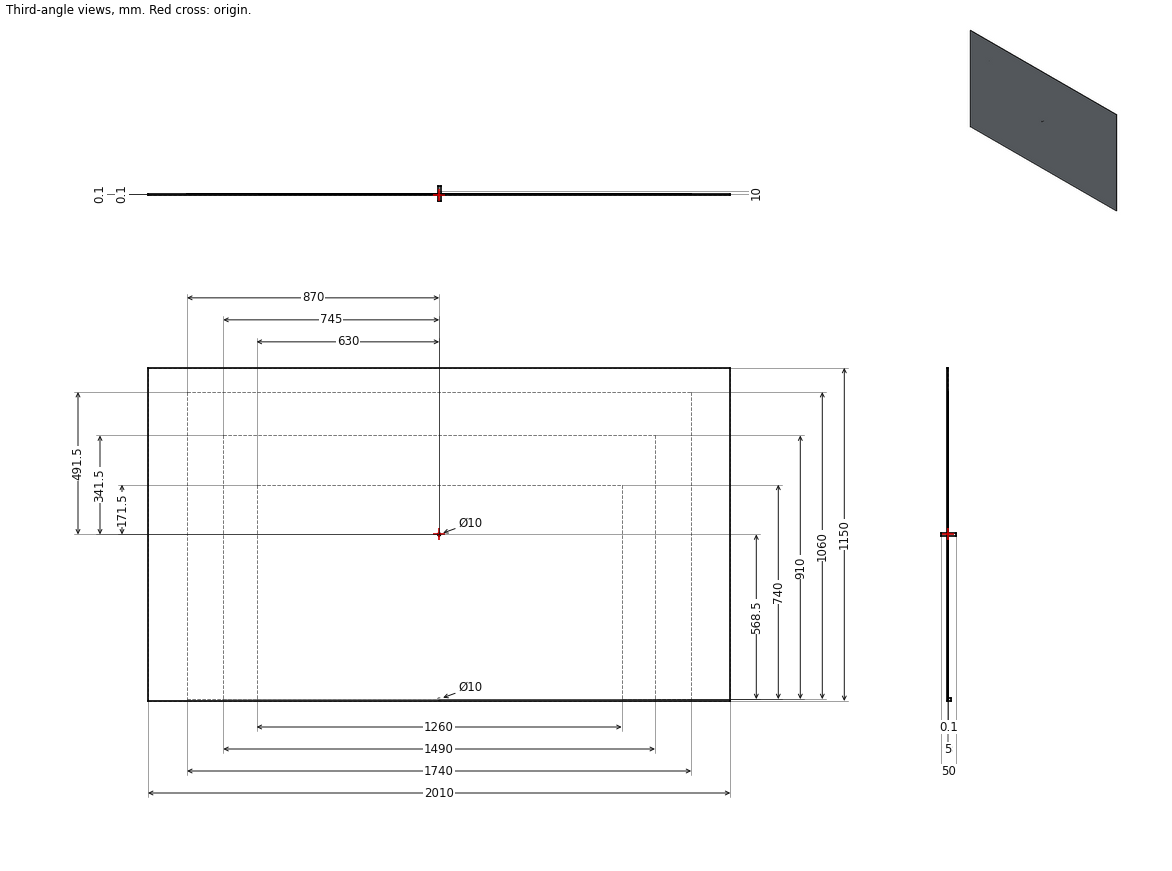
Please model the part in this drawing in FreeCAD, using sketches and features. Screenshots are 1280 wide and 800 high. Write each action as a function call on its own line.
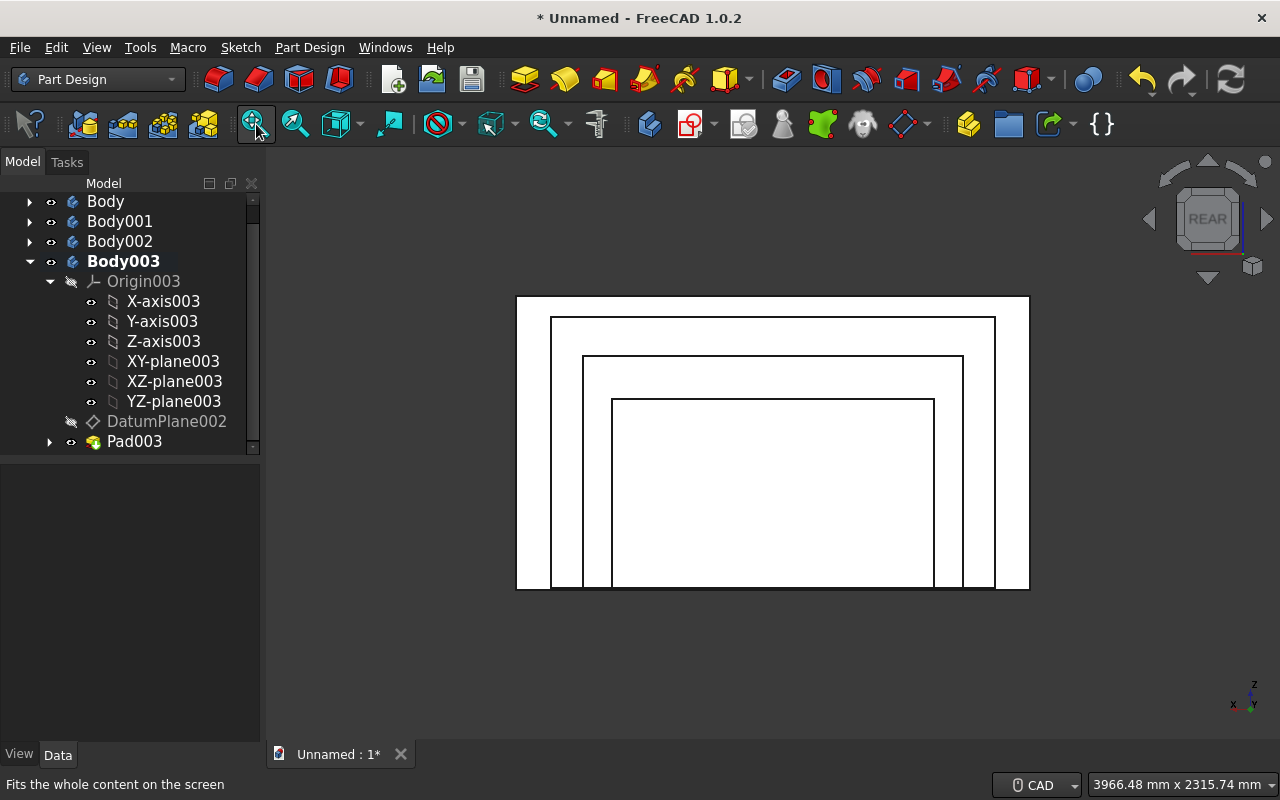
click(256, 124)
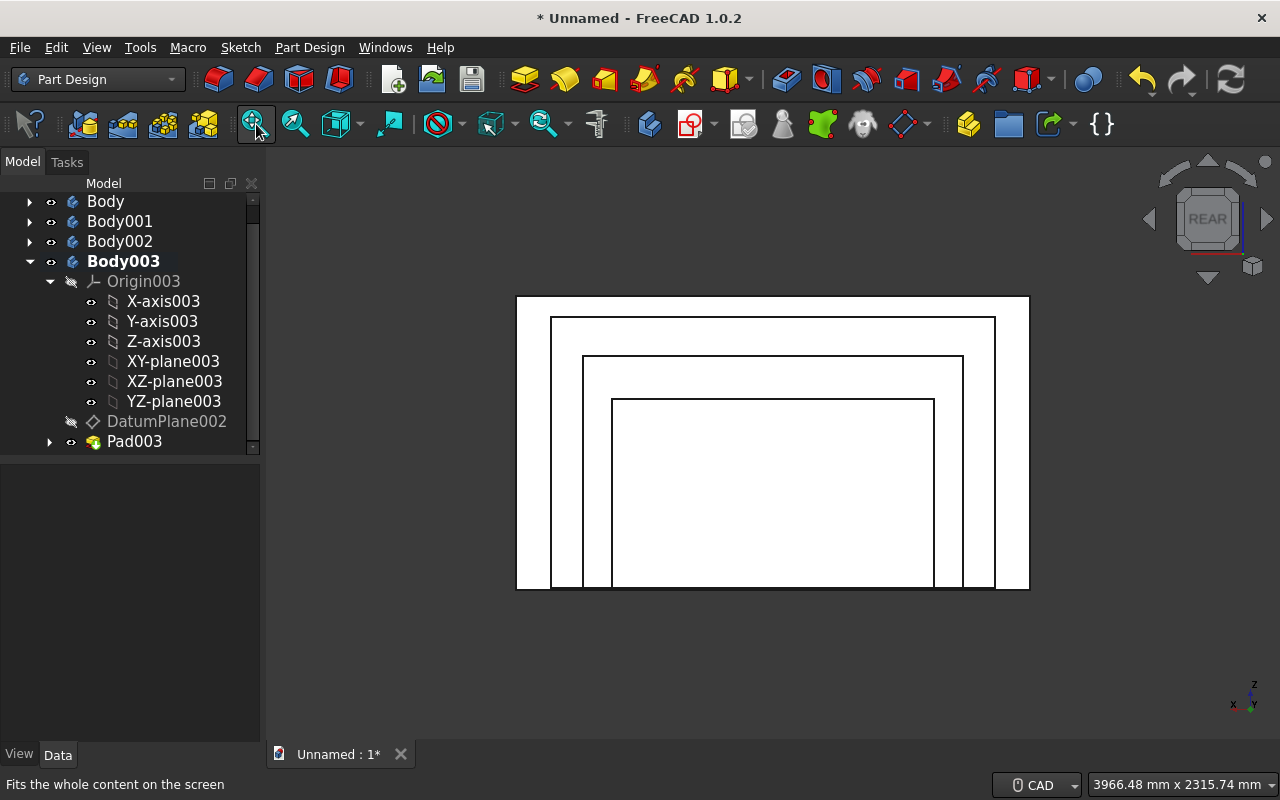
click(727, 493)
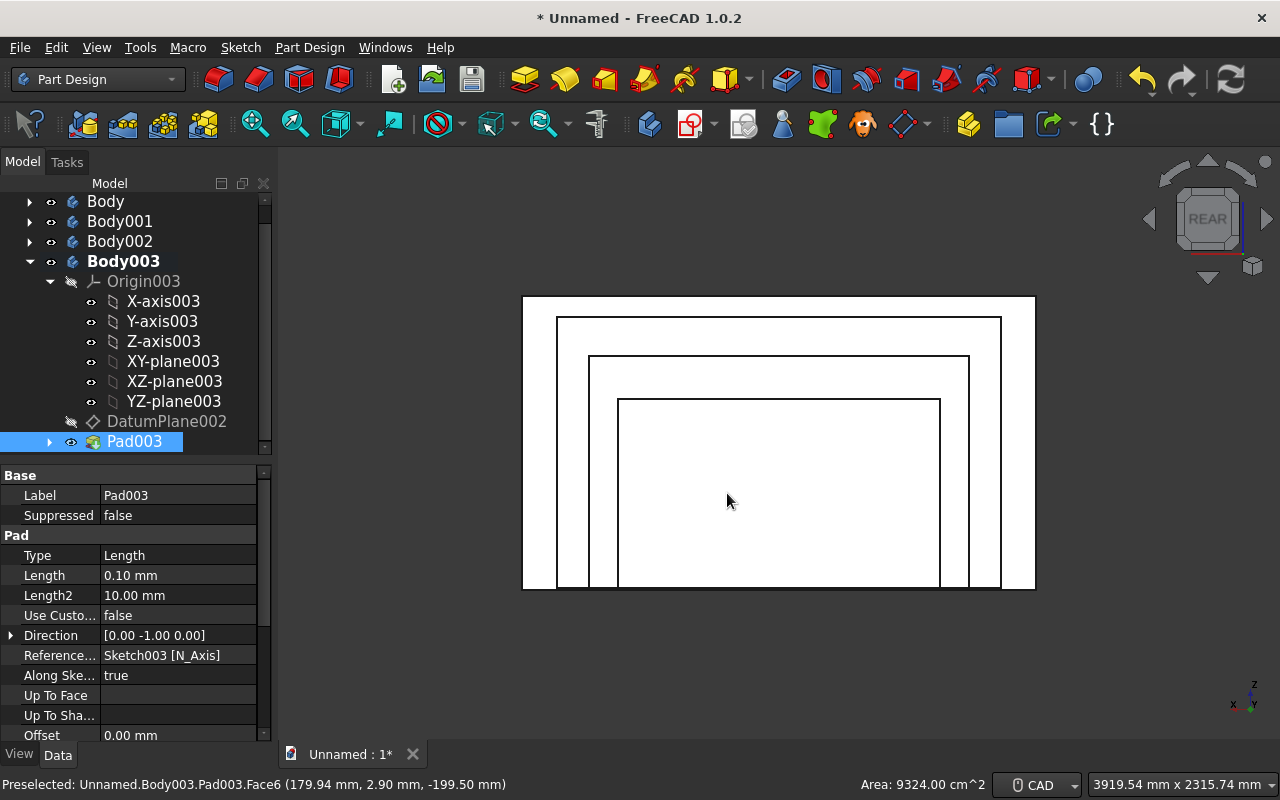
click(690, 124)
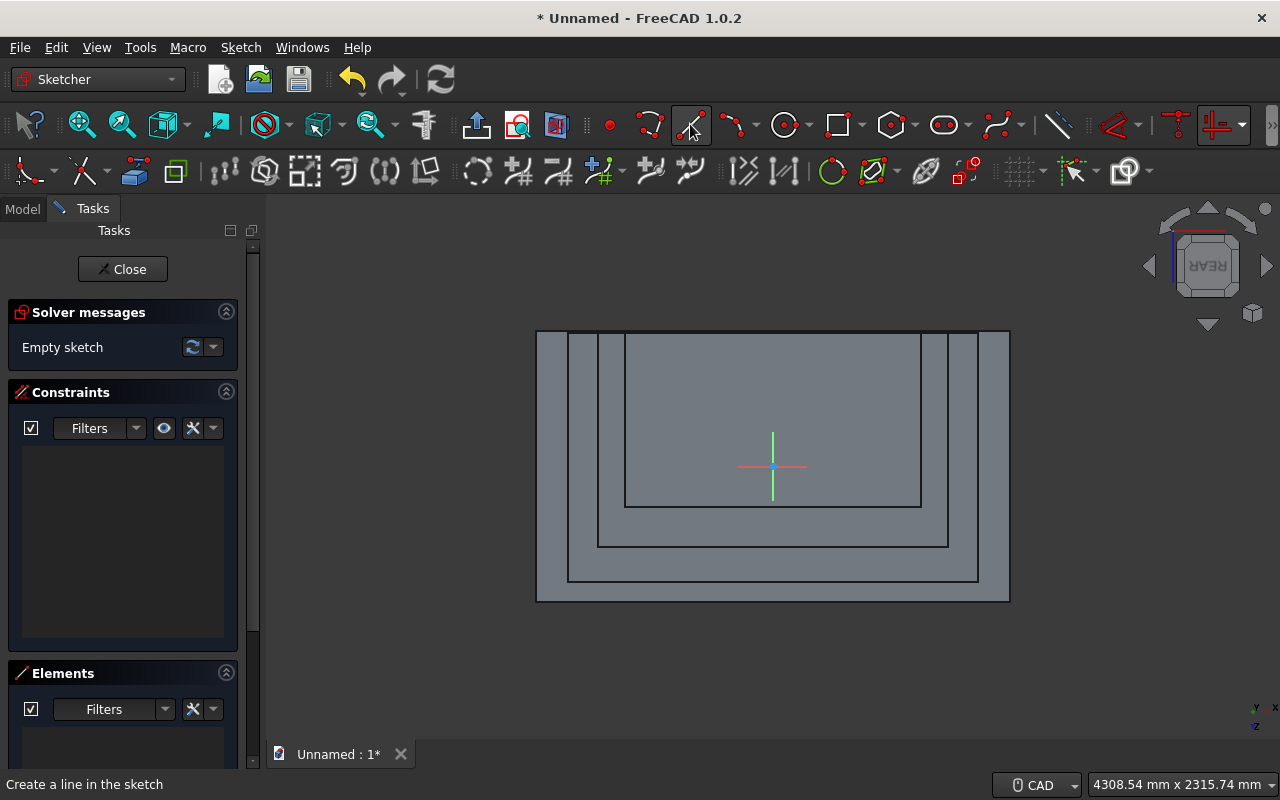
scroll(777, 466, up, 15)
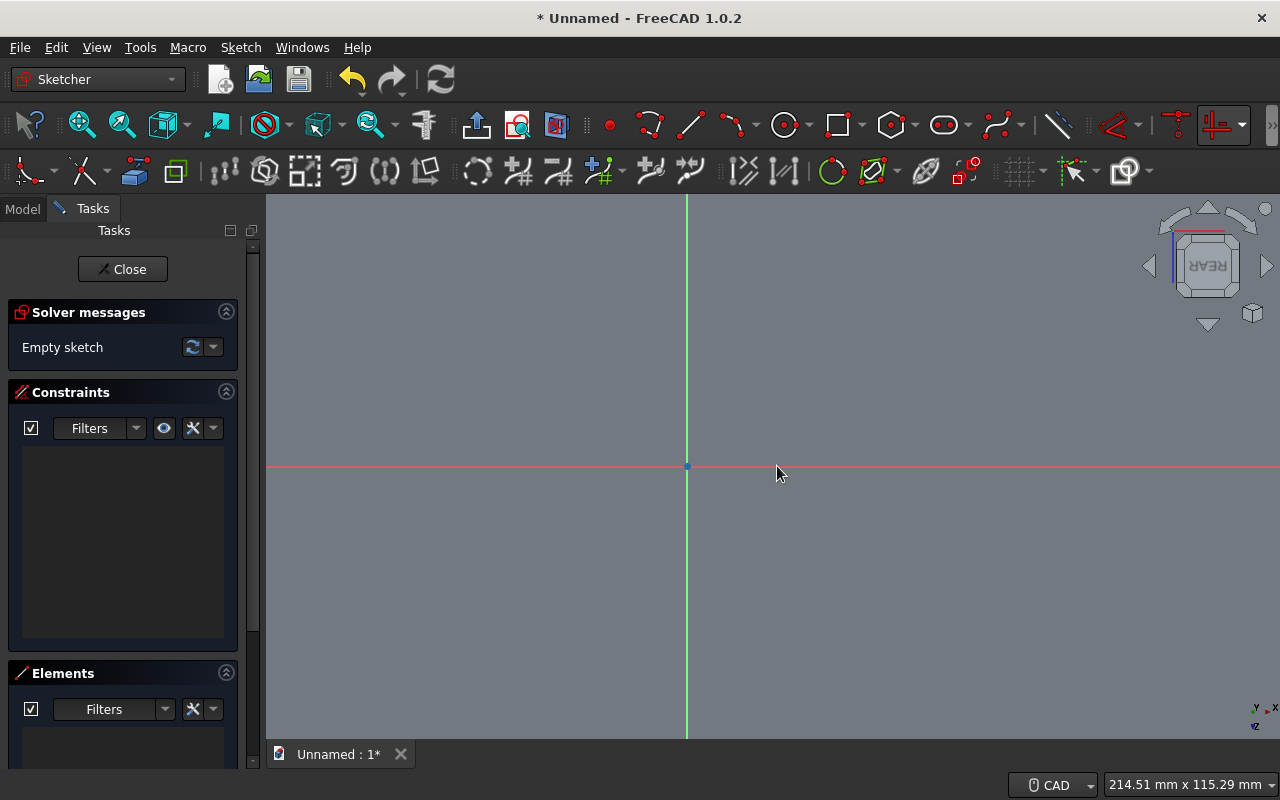
scroll(684, 466, up, 10)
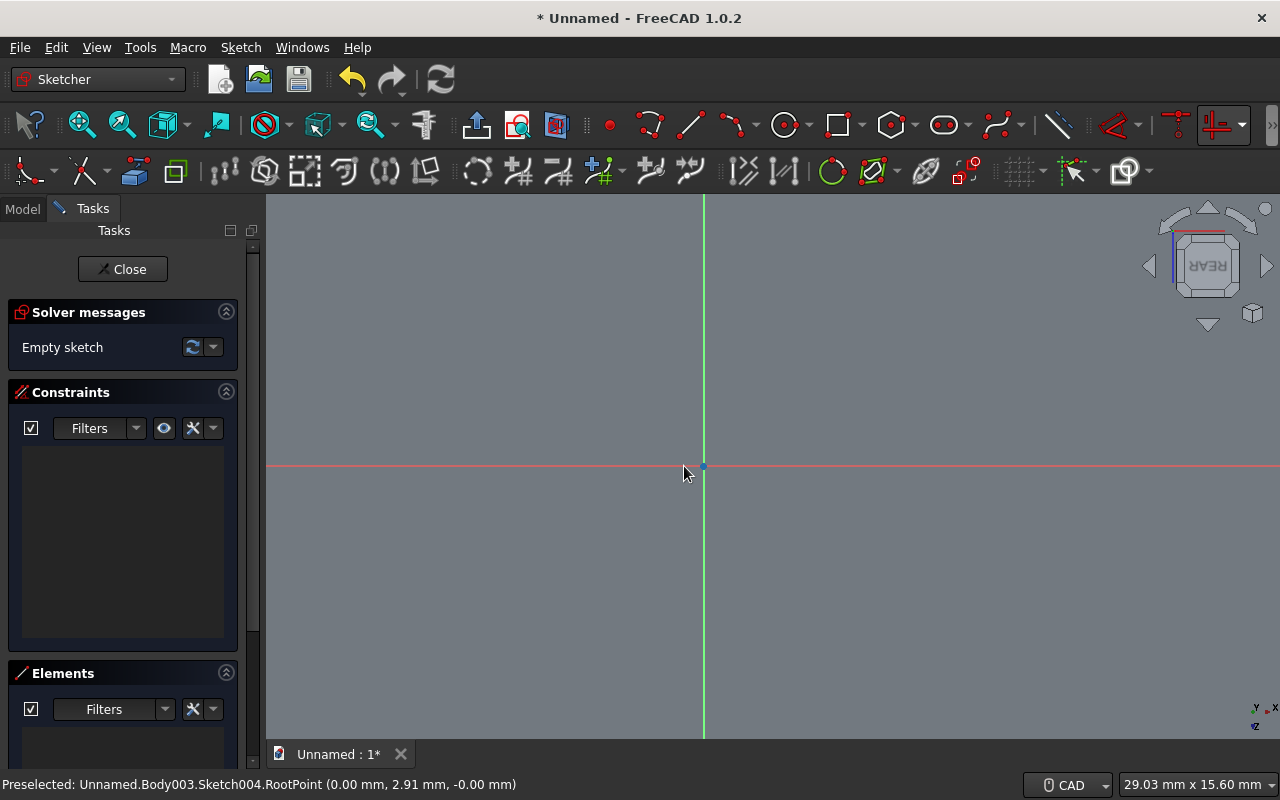
click(786, 126)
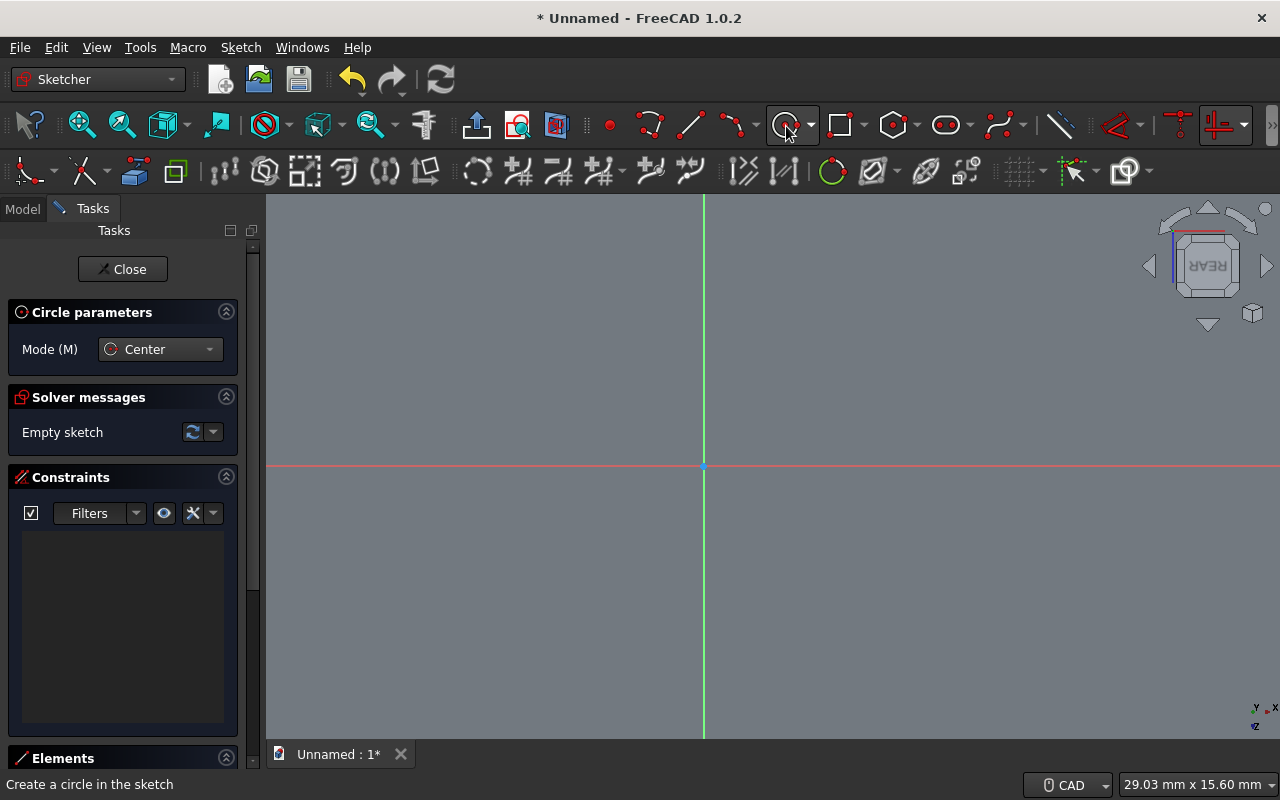
click(704, 466)
move(827, 343)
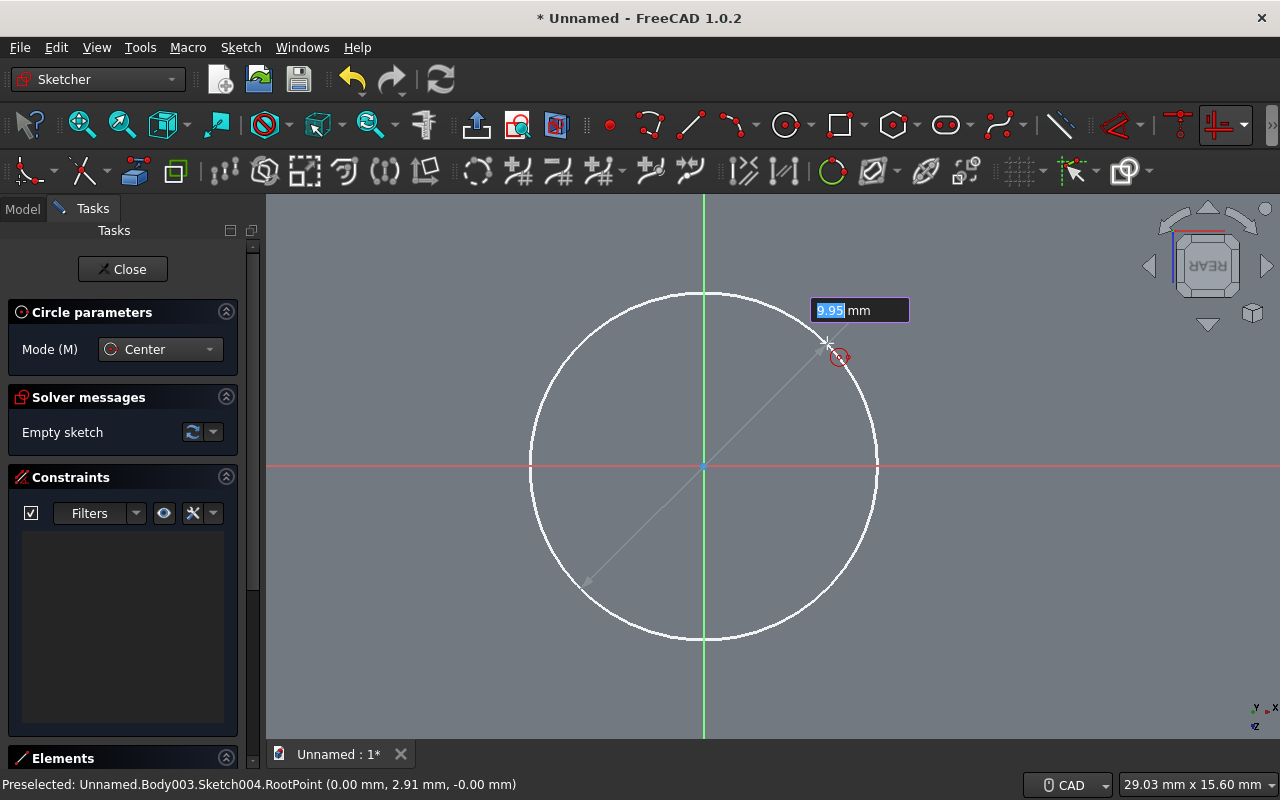
text(10)
key(Return)
key(Escape)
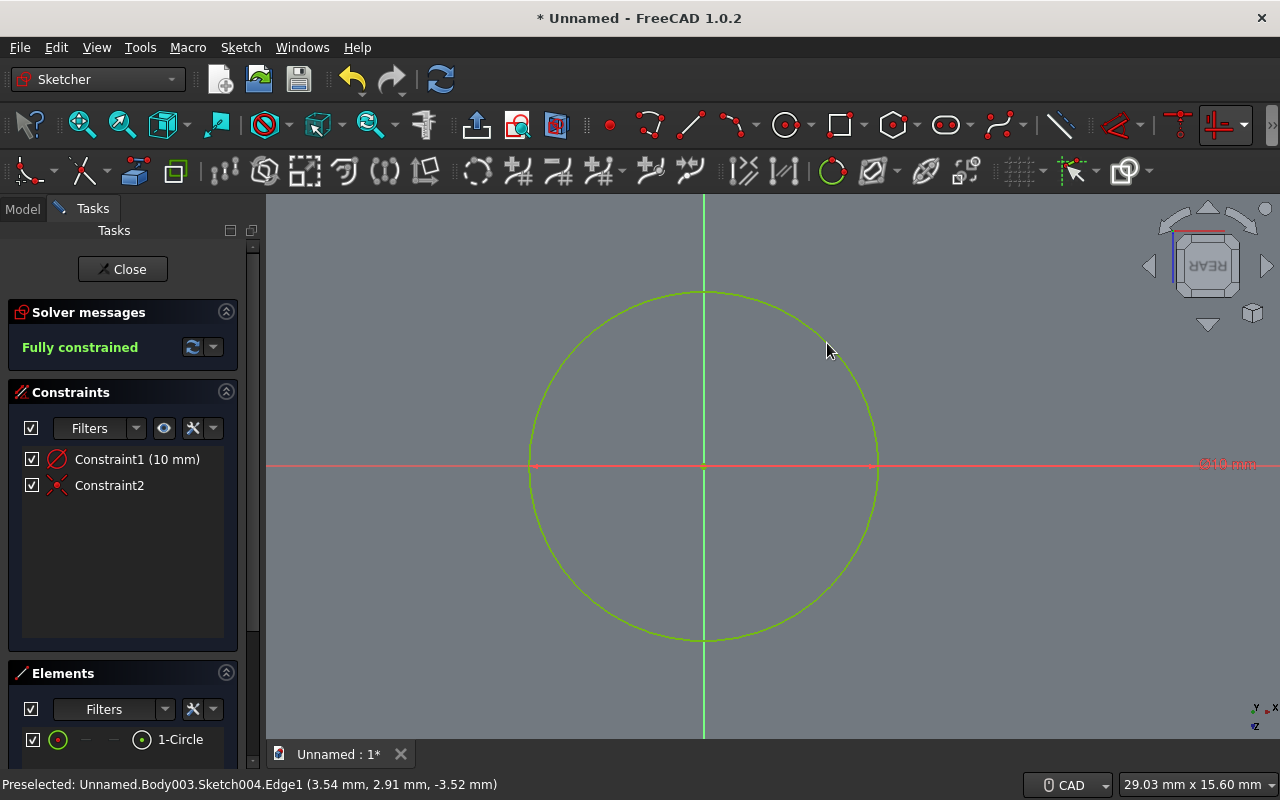
click(123, 269)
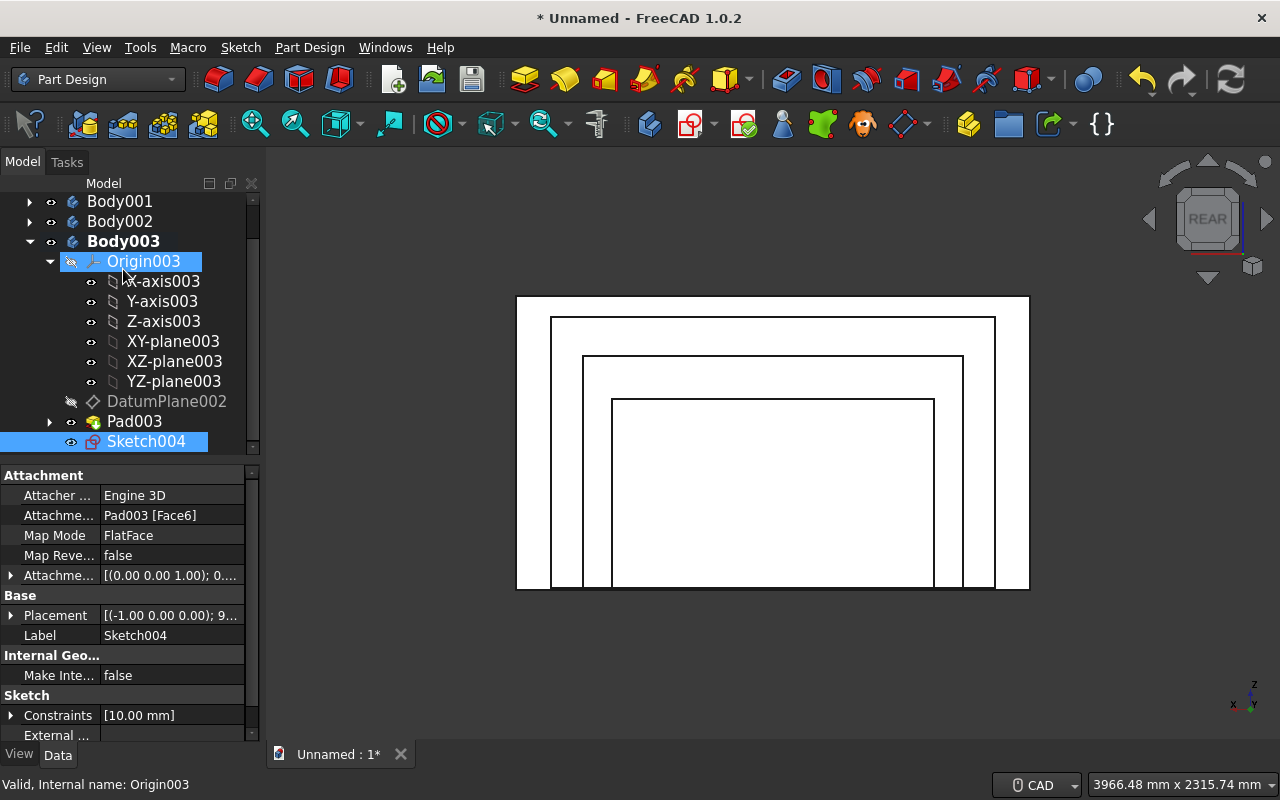
click(526, 80)